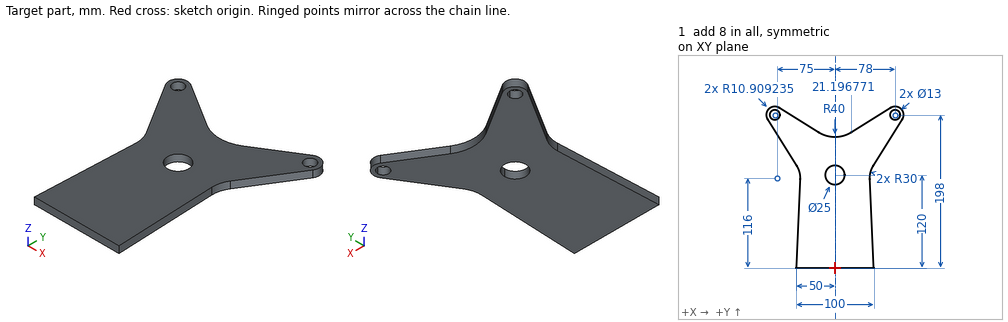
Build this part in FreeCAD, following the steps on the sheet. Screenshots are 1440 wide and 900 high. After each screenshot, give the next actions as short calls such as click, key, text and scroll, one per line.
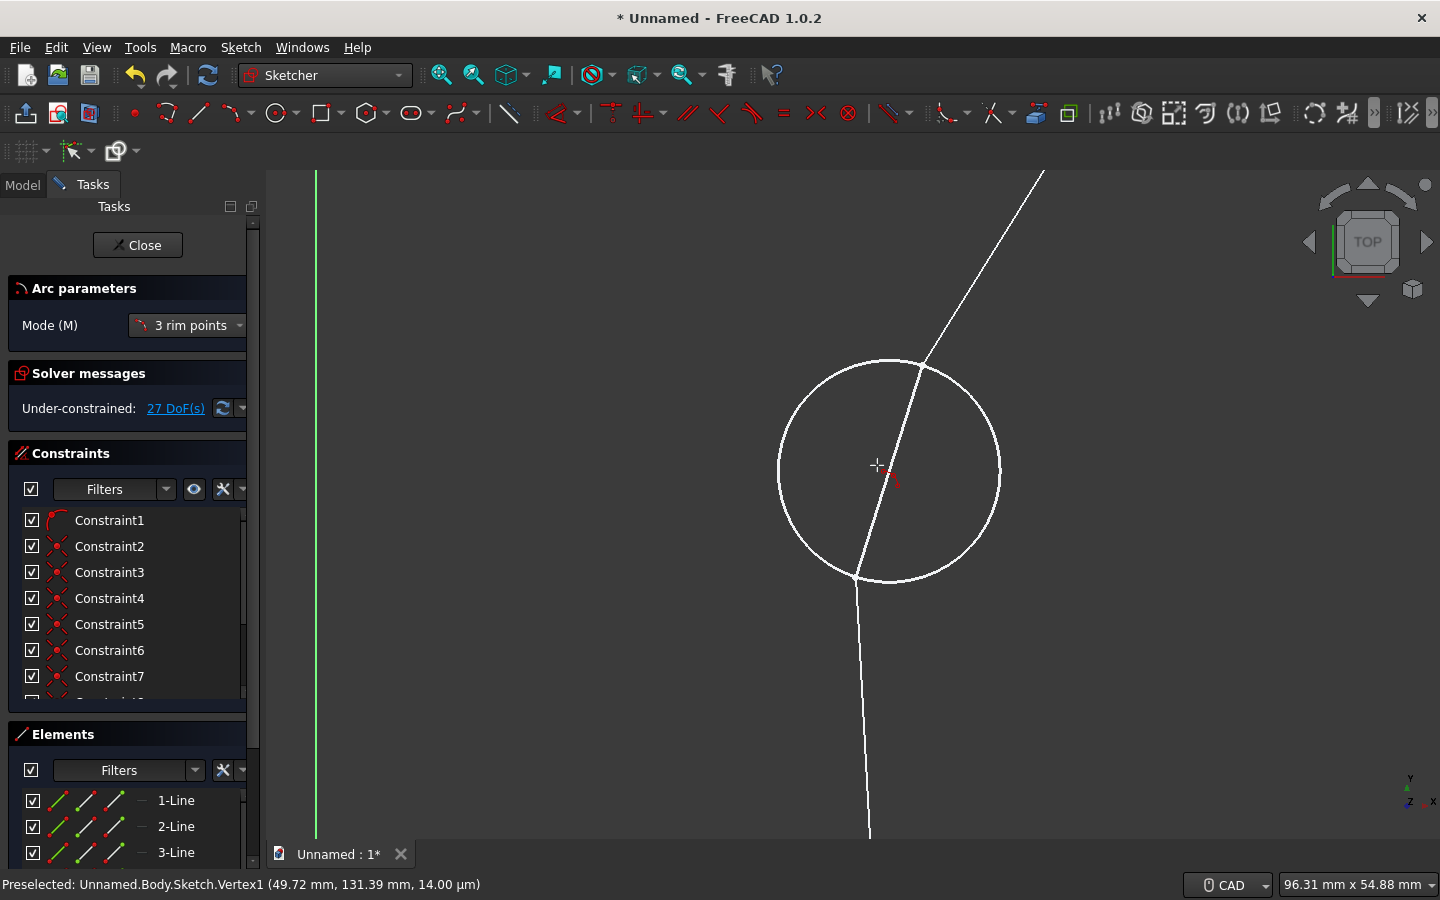
click(877, 460)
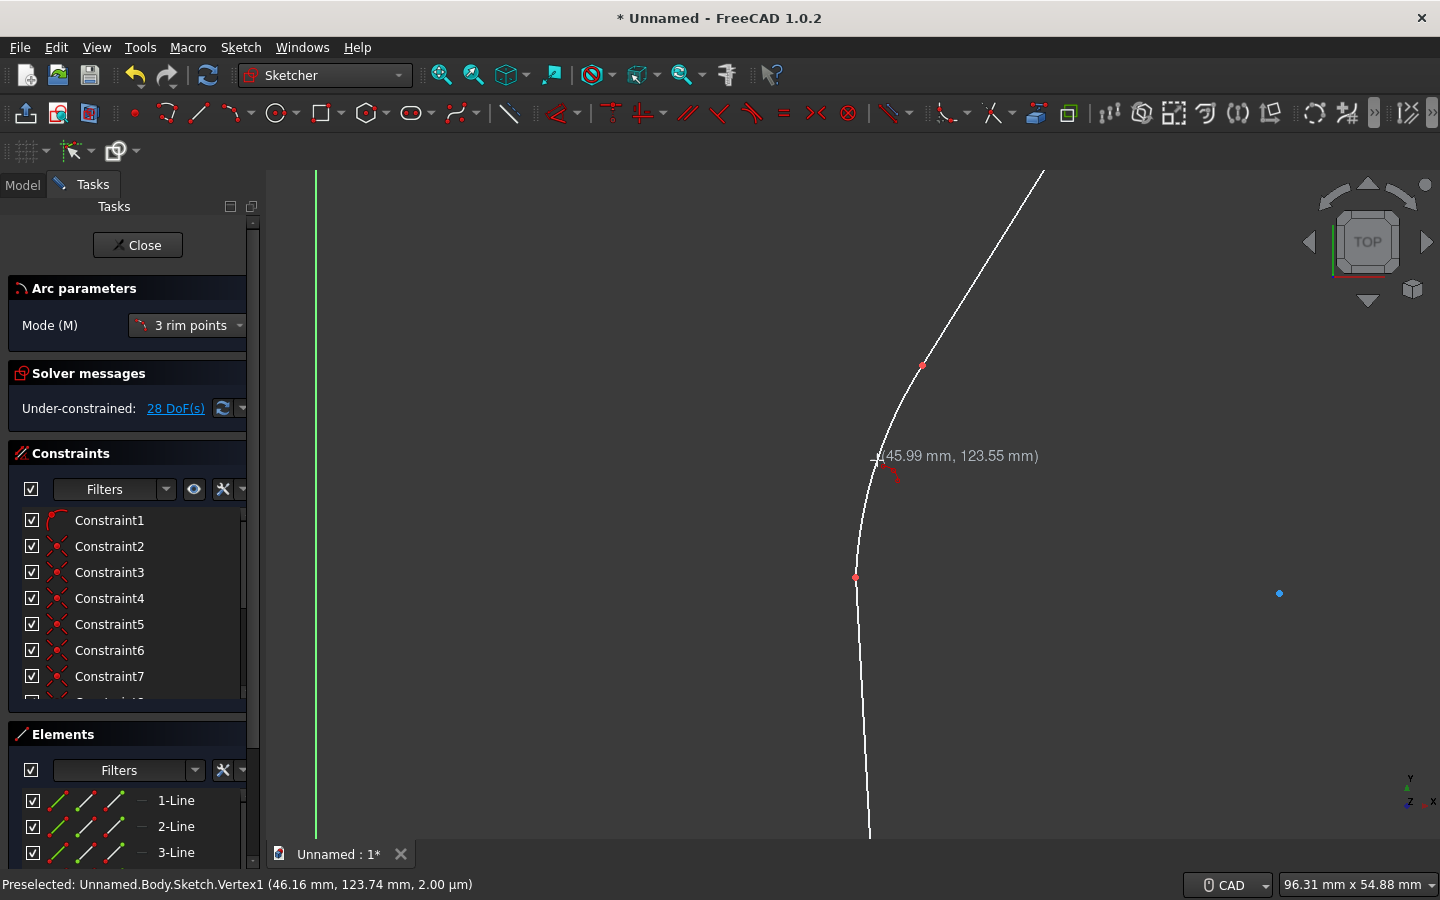
click(276, 114)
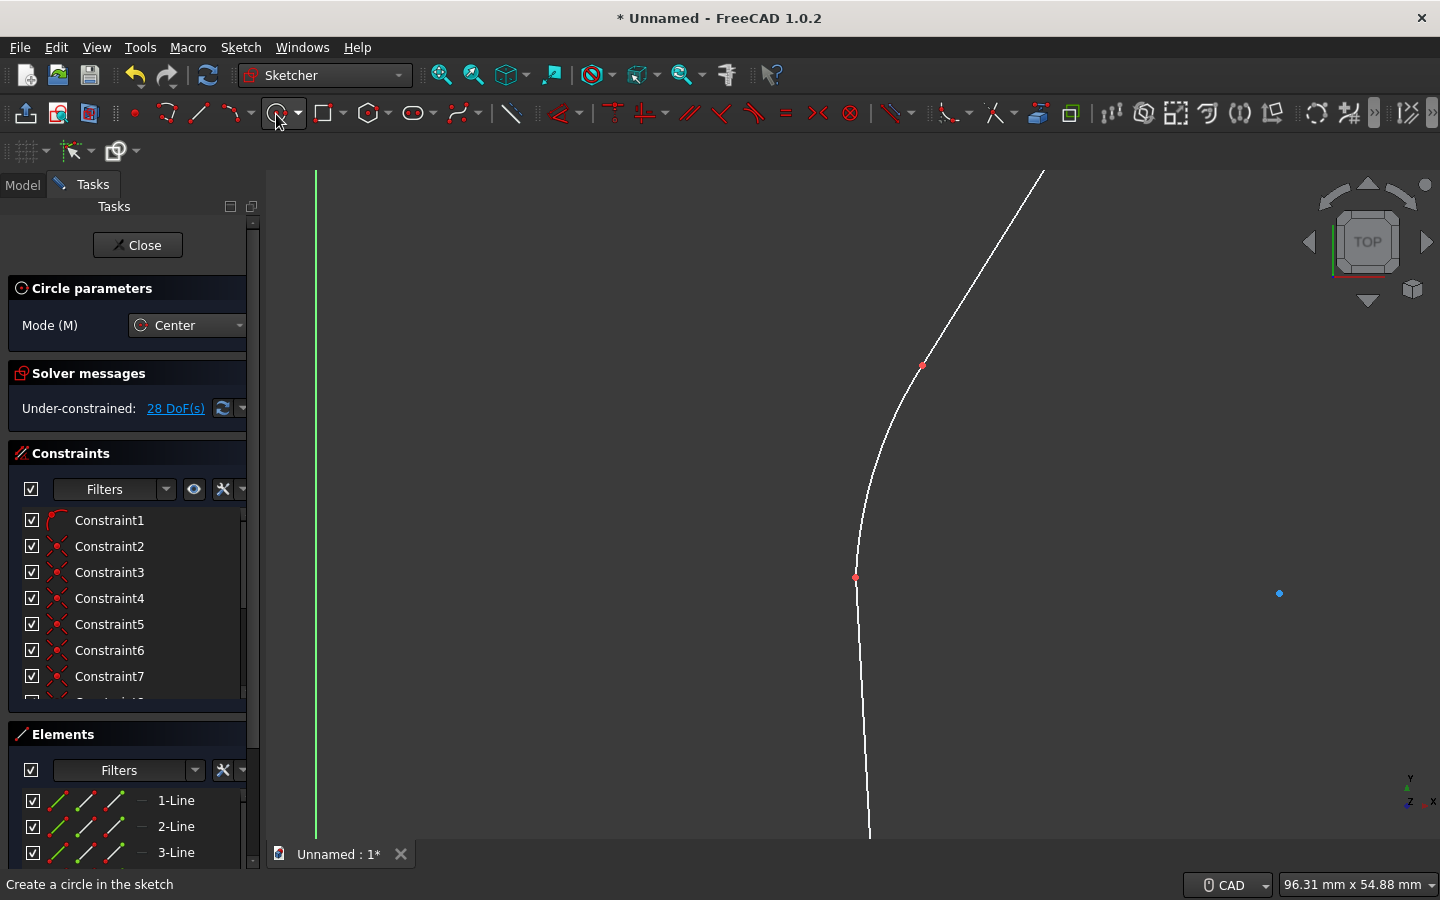
scroll(877, 465, down, 9)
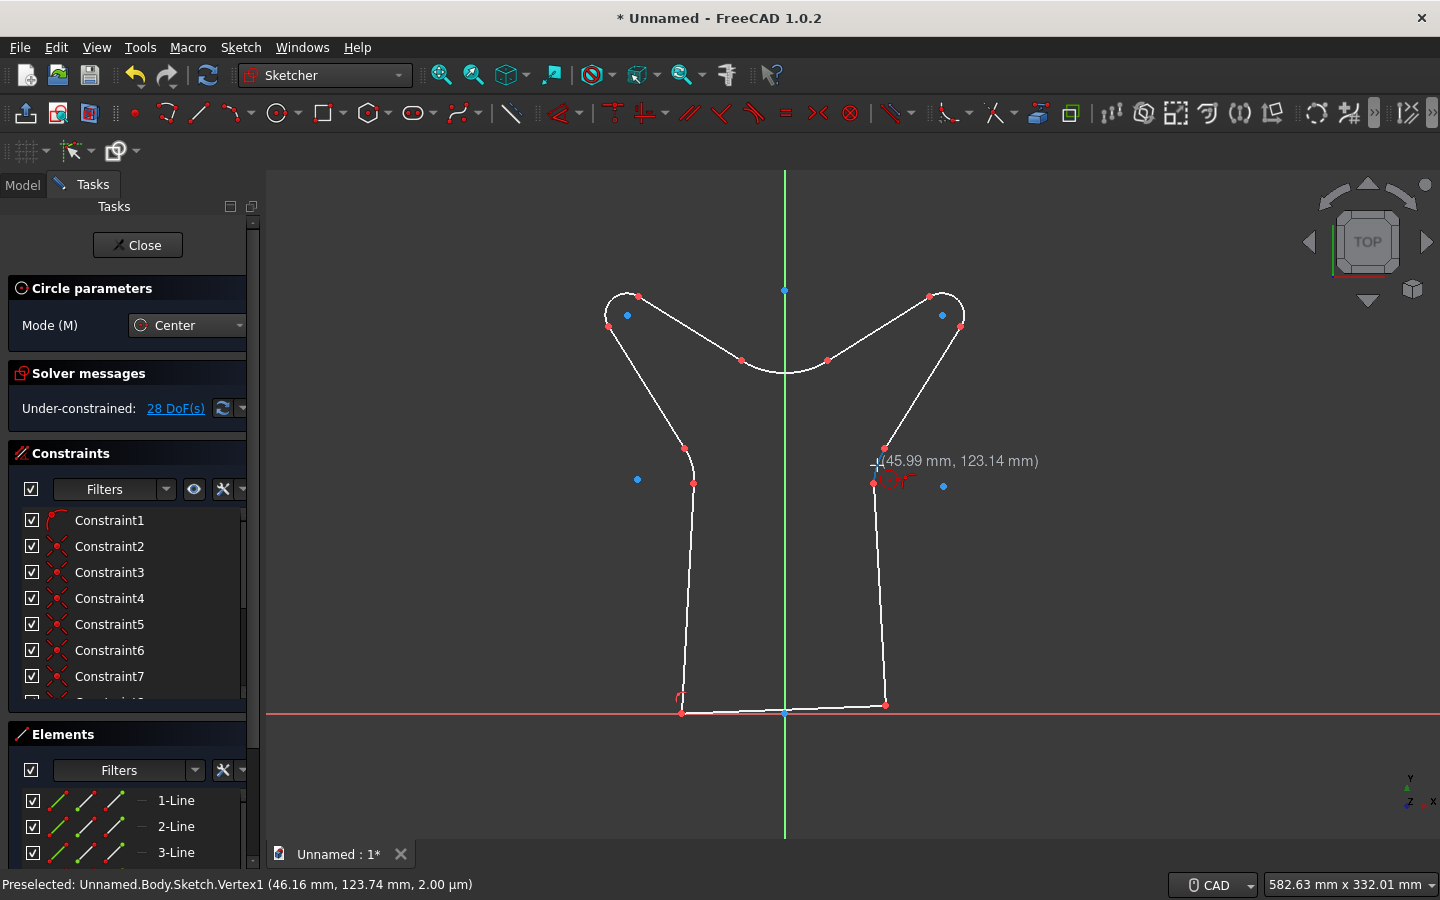
click(785, 472)
move(803, 454)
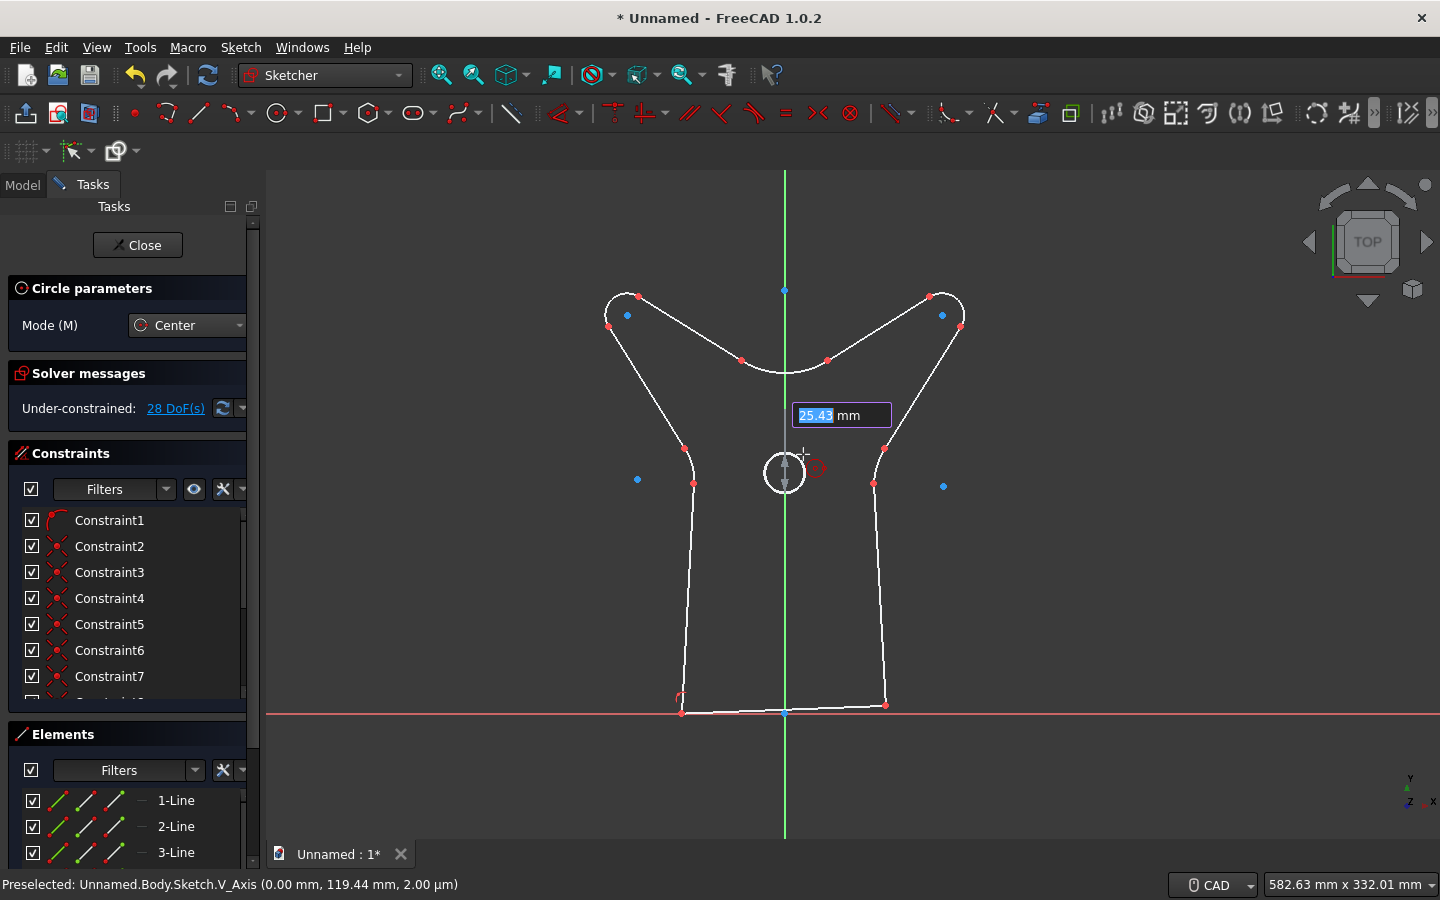
text(25)
key(Return)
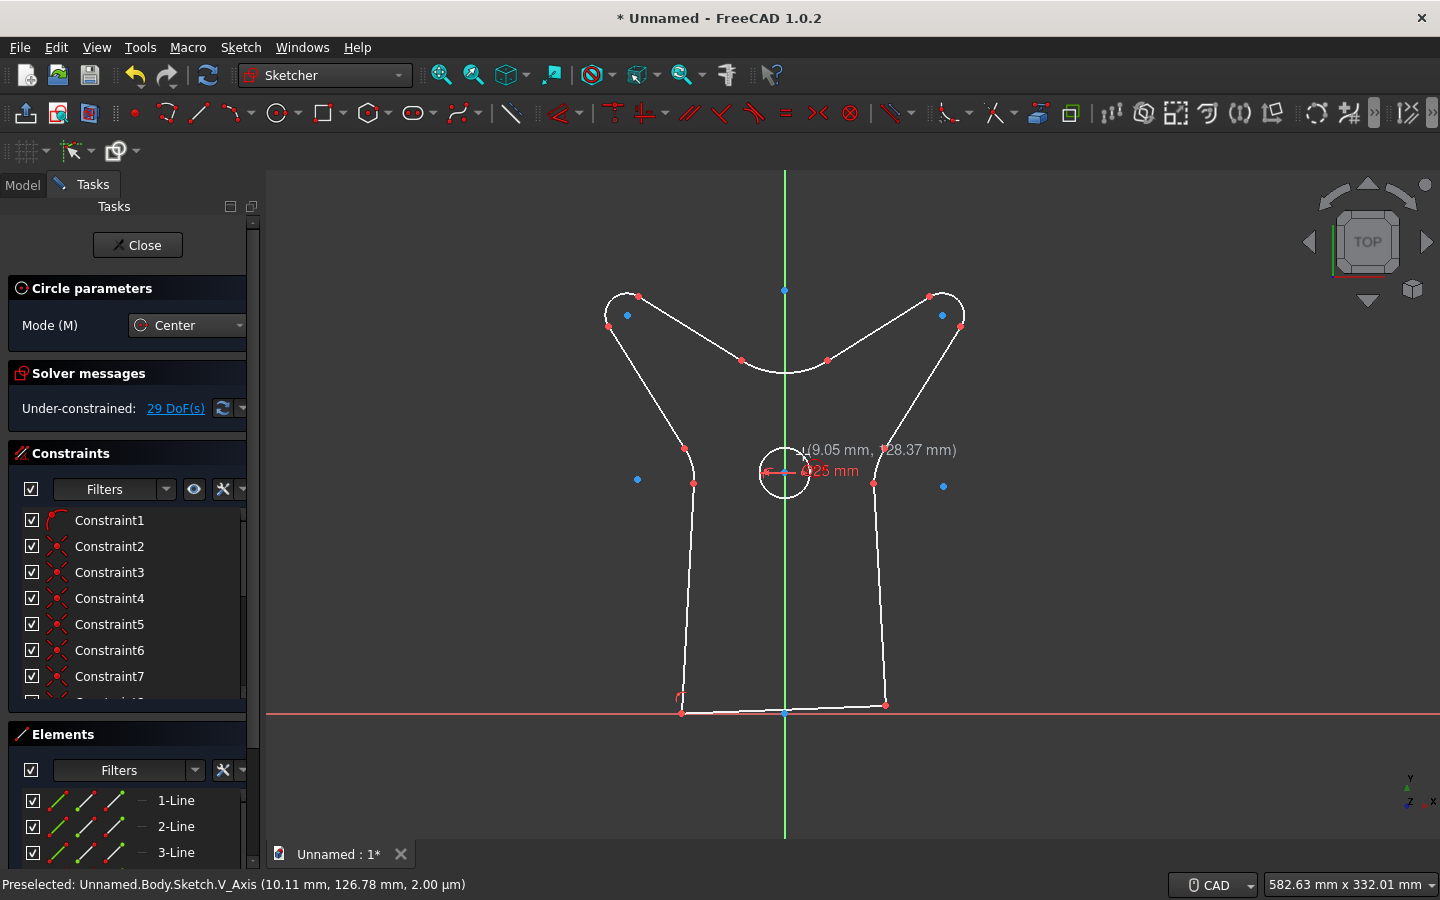
scroll(942, 315, up, 3)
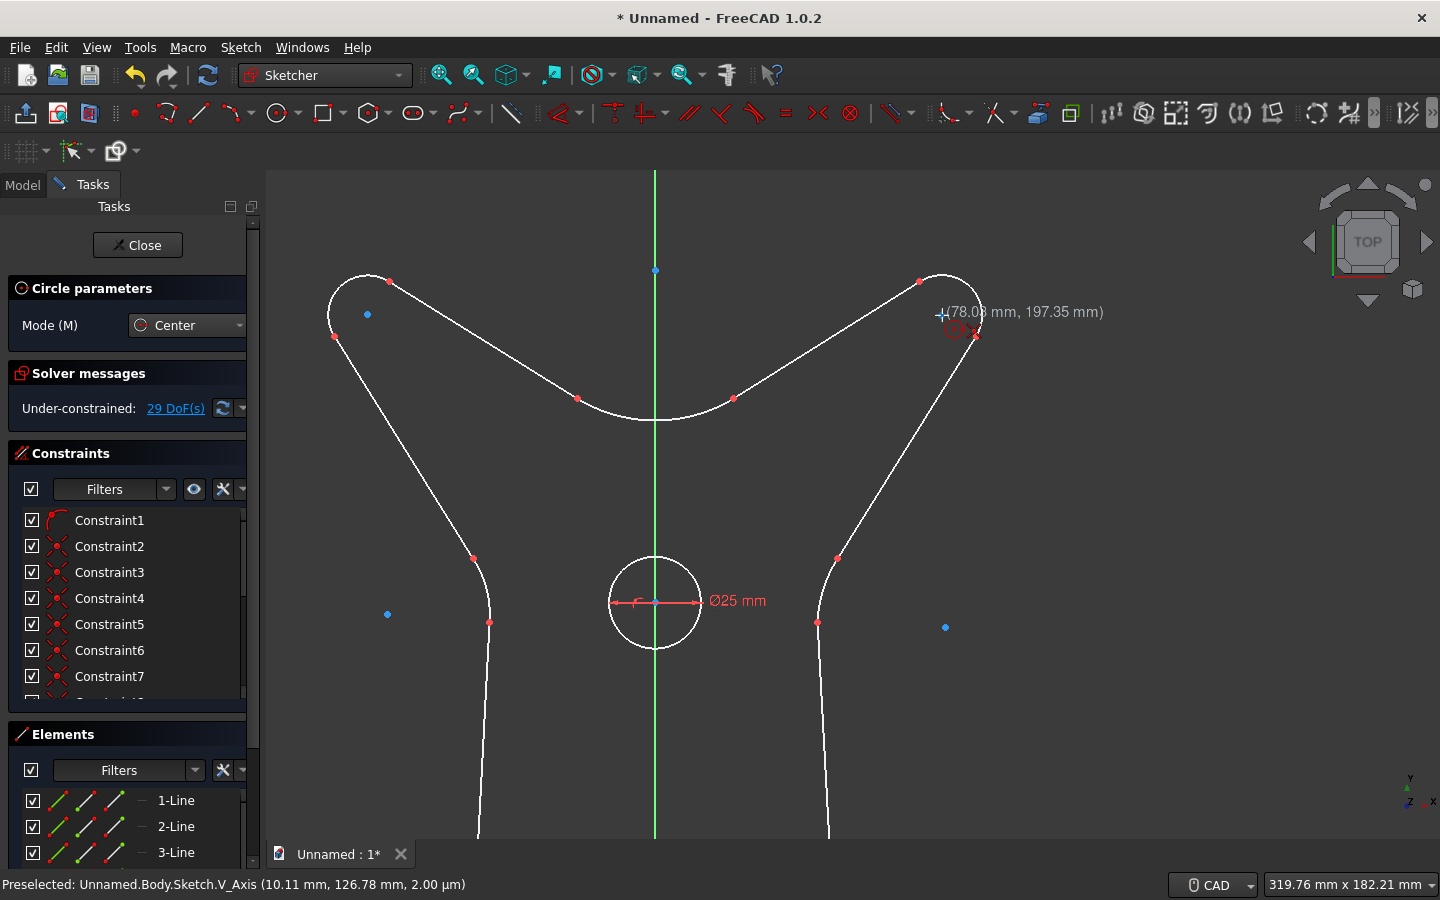
click(941, 314)
move(958, 297)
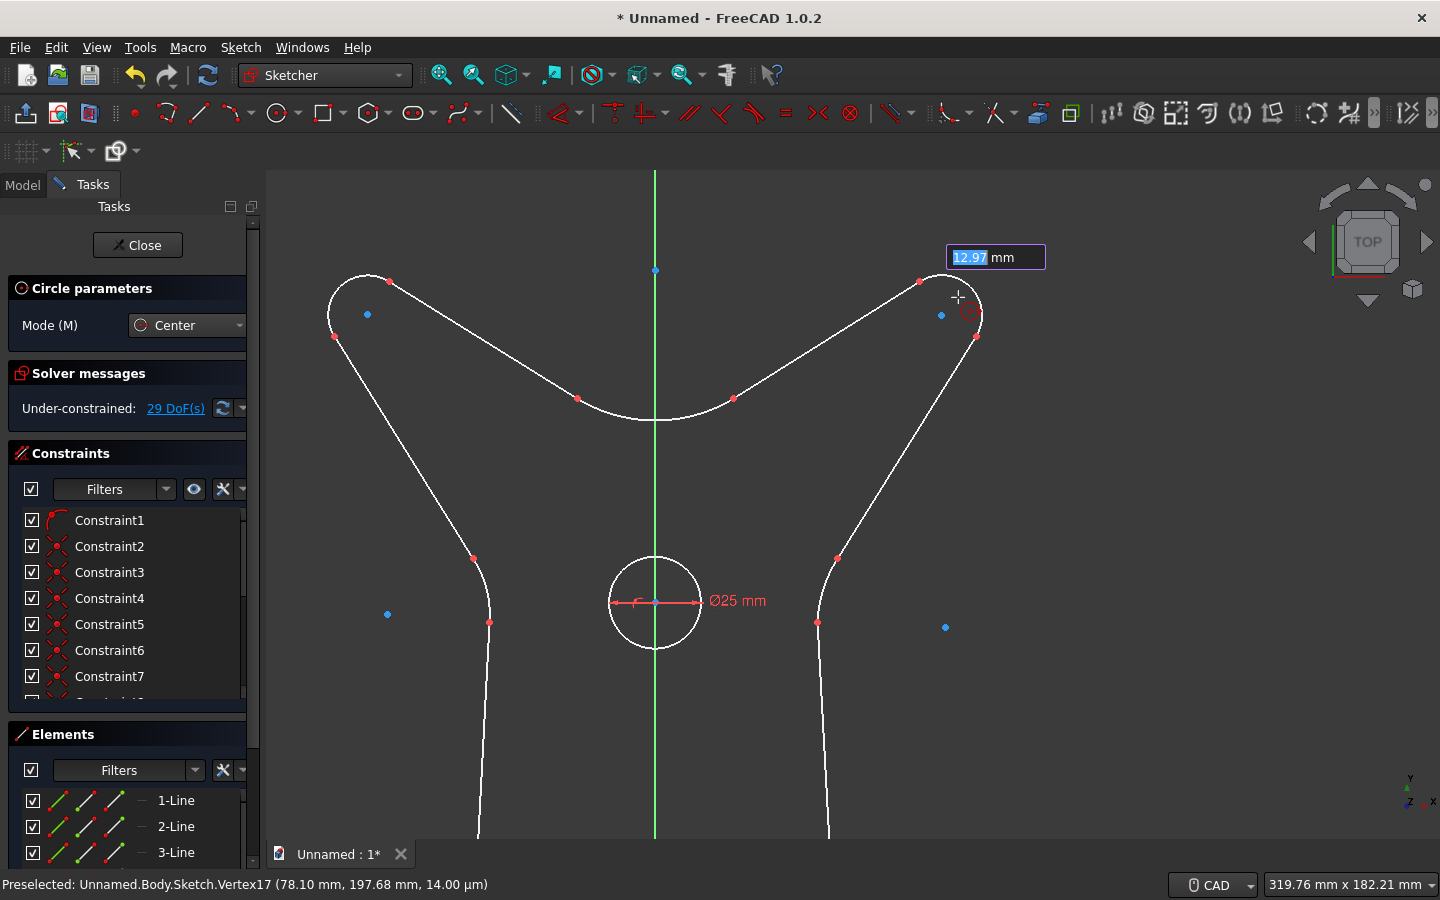
text(13)
key(Return)